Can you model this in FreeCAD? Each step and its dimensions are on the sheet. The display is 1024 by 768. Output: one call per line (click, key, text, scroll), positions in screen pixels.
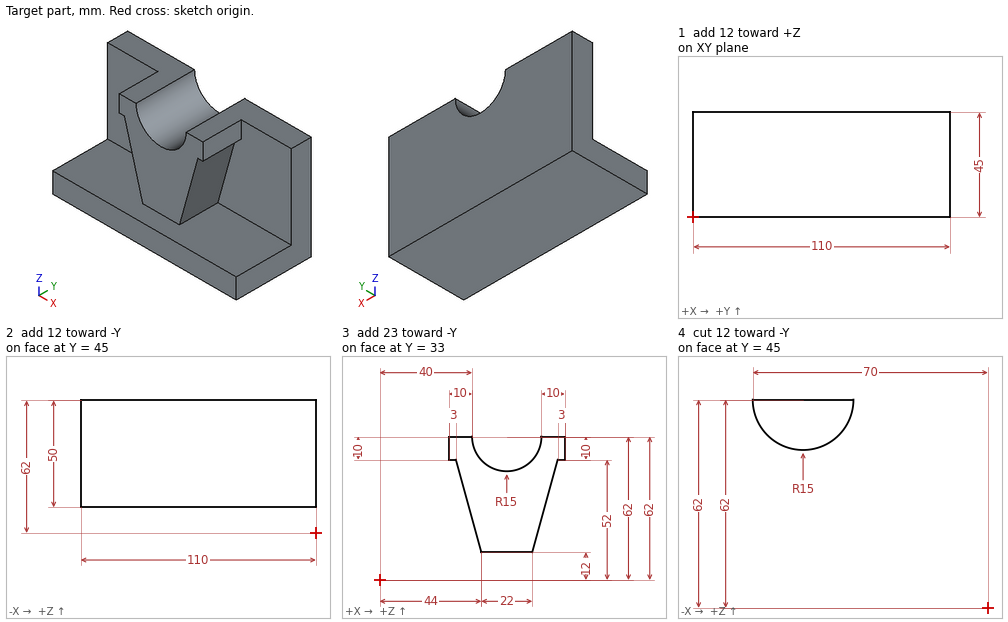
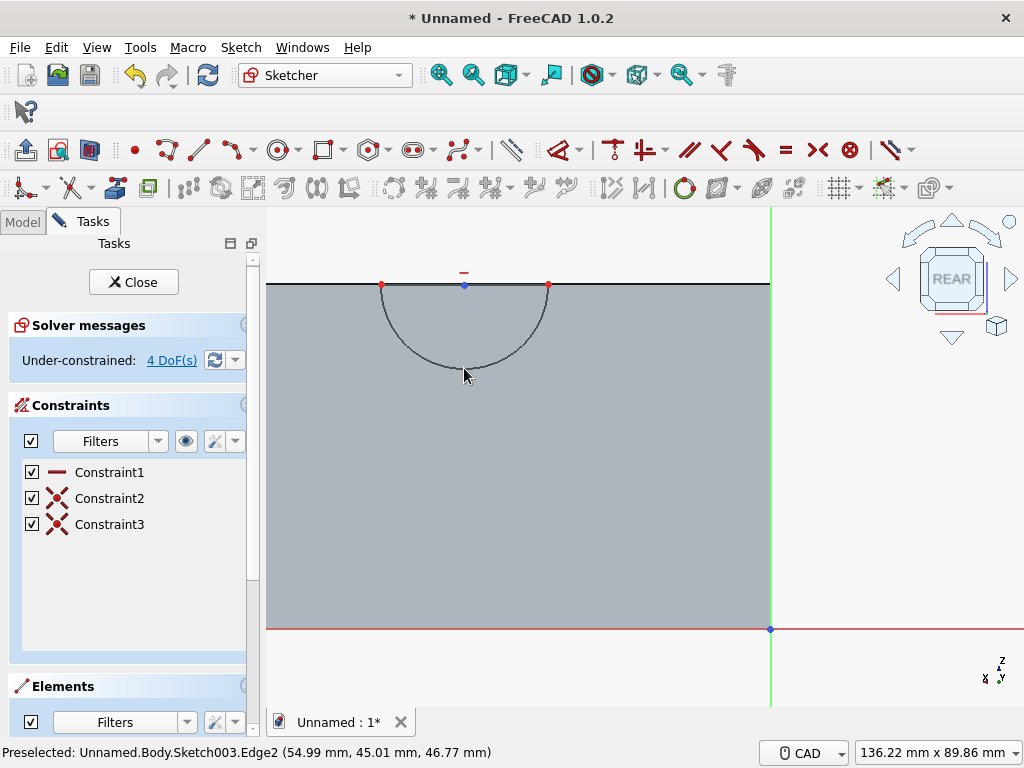
click(558, 150)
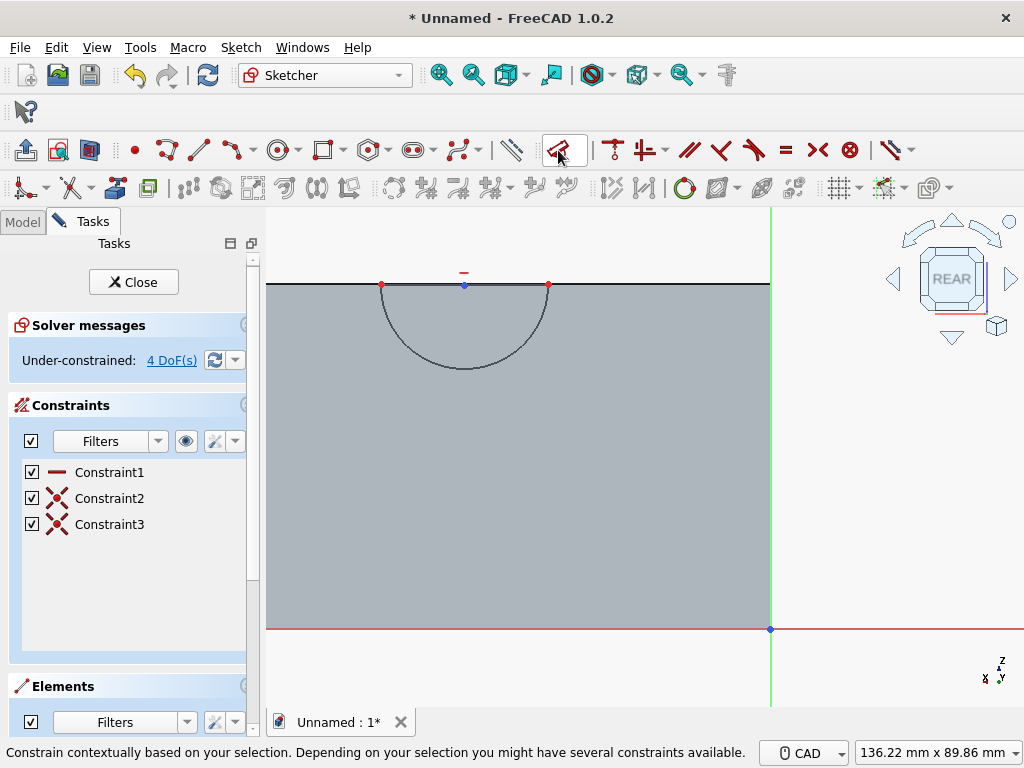
click(415, 353)
click(396, 379)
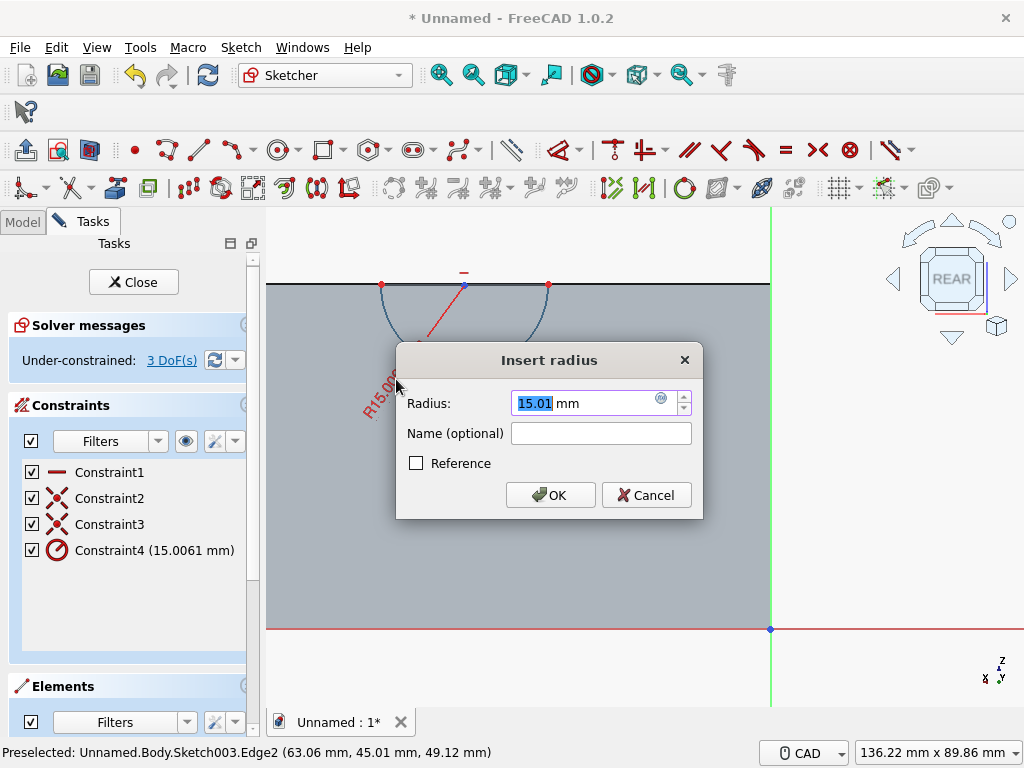
text(15)
key(Return)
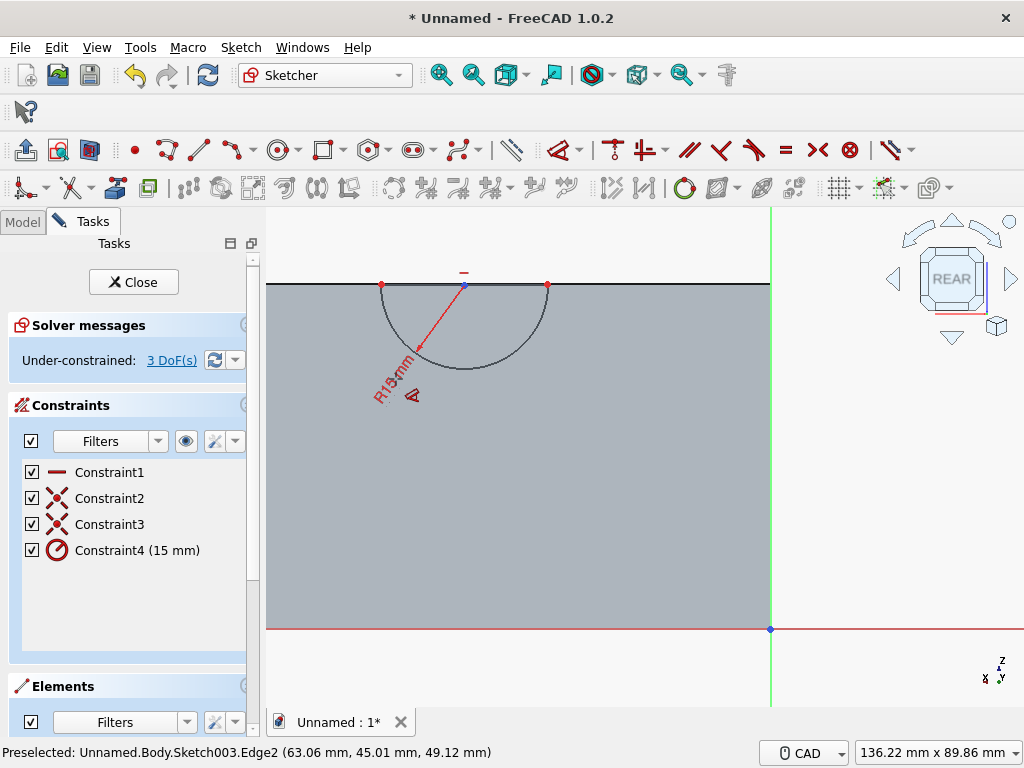
click(381, 285)
click(576, 663)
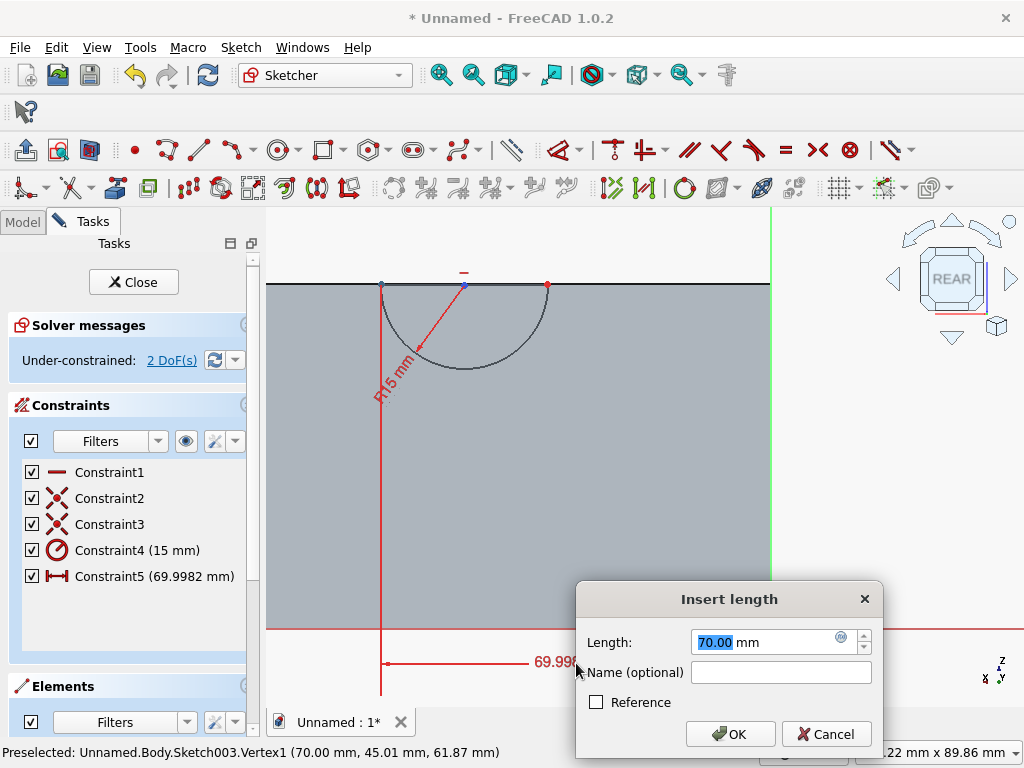
text(70)
key(Return)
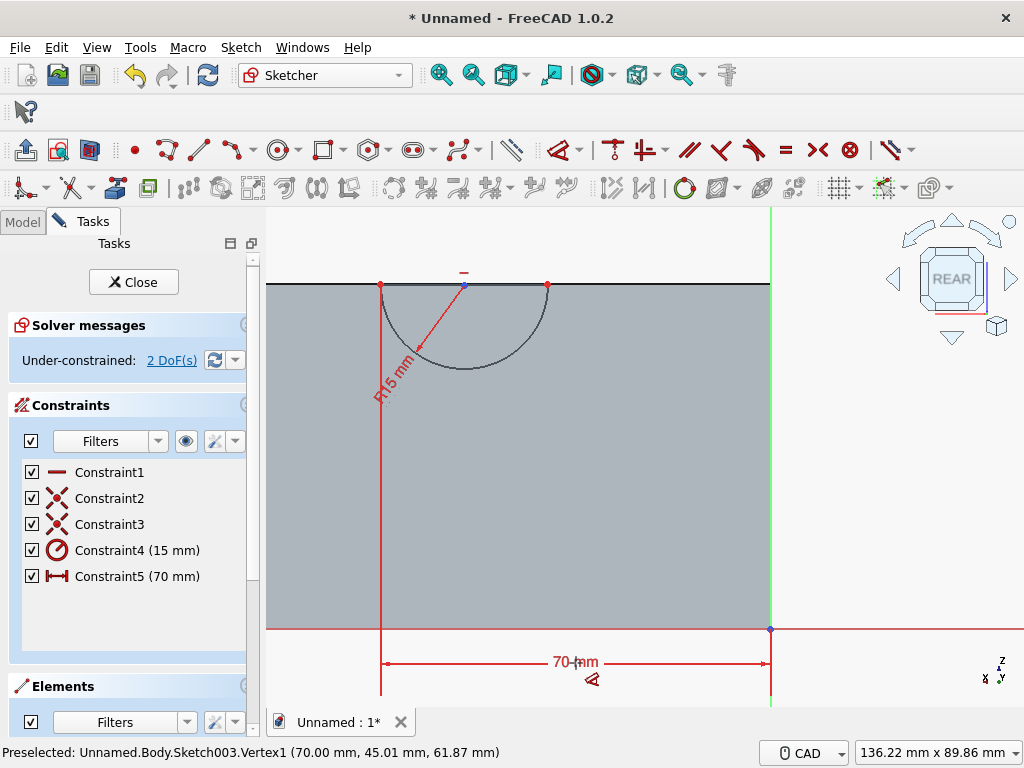
click(381, 285)
click(805, 457)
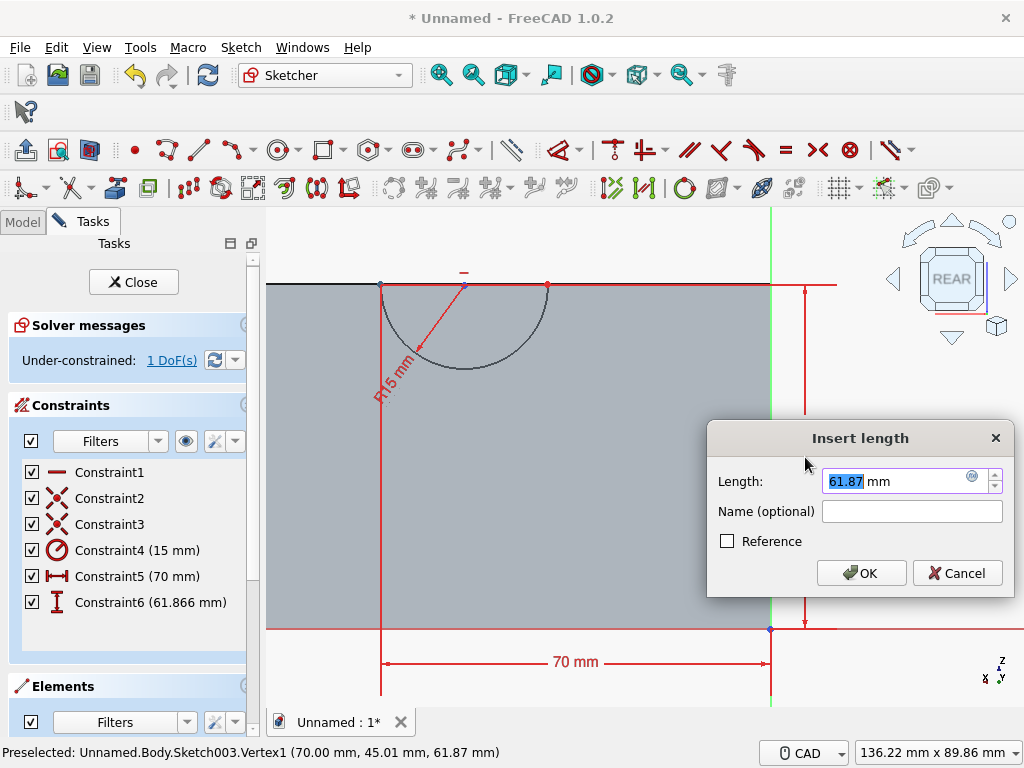
text(62)
key(Return)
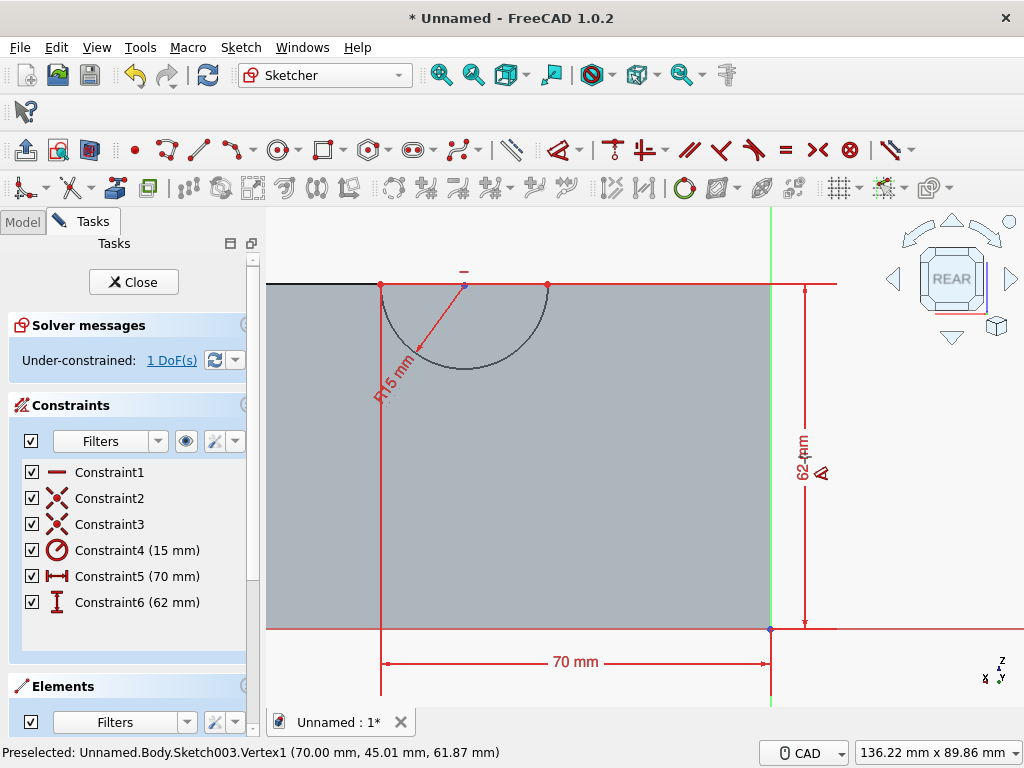
click(464, 285)
click(805, 378)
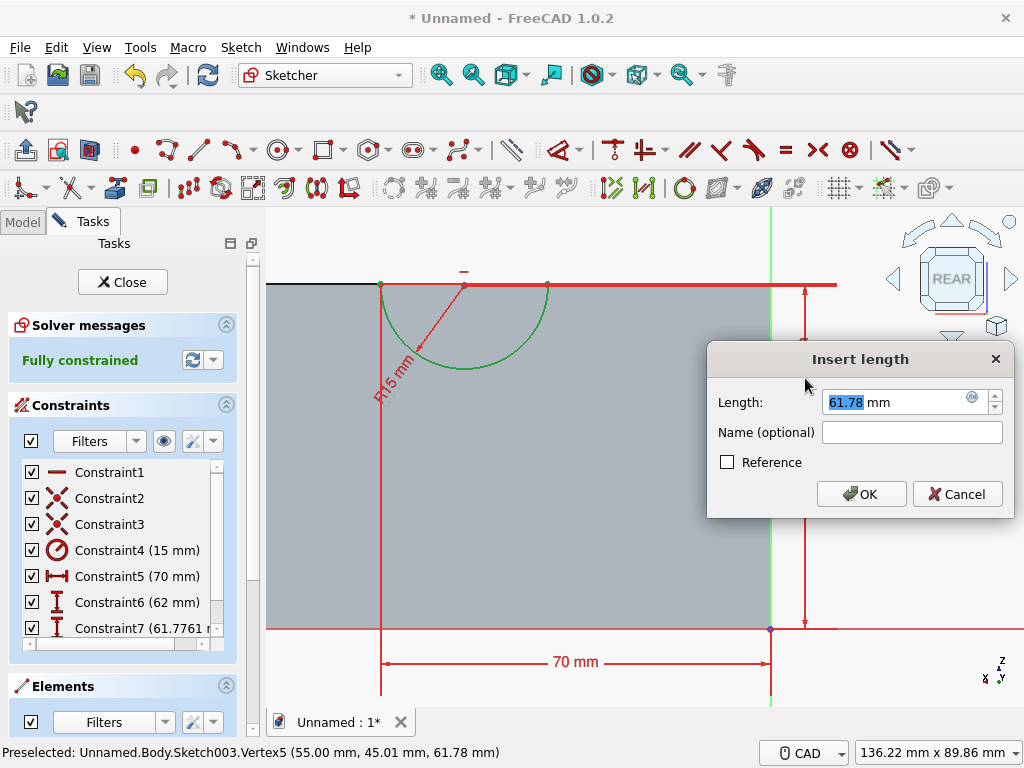
text(62)
key(Return)
key(Escape)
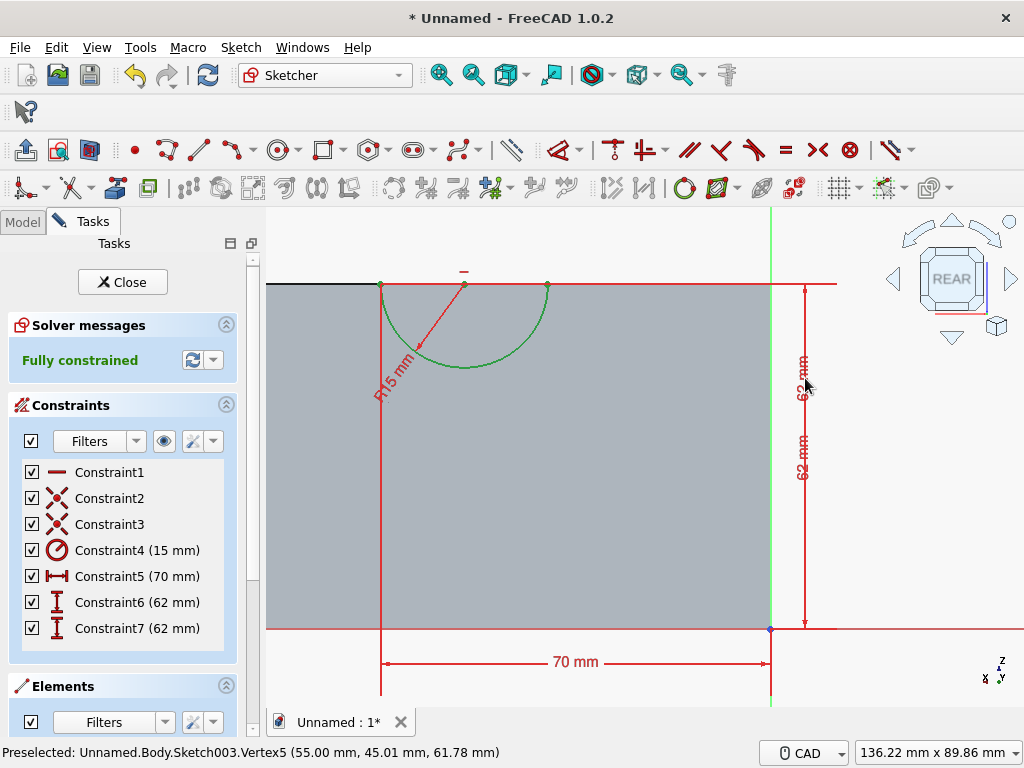
click(123, 282)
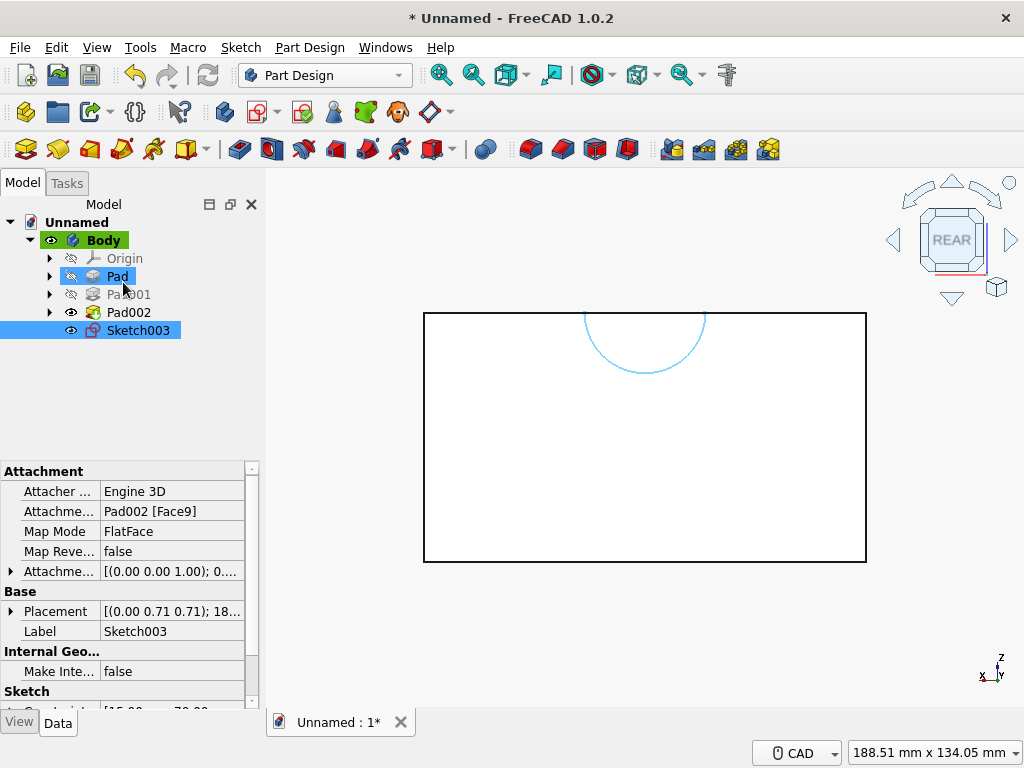
click(240, 150)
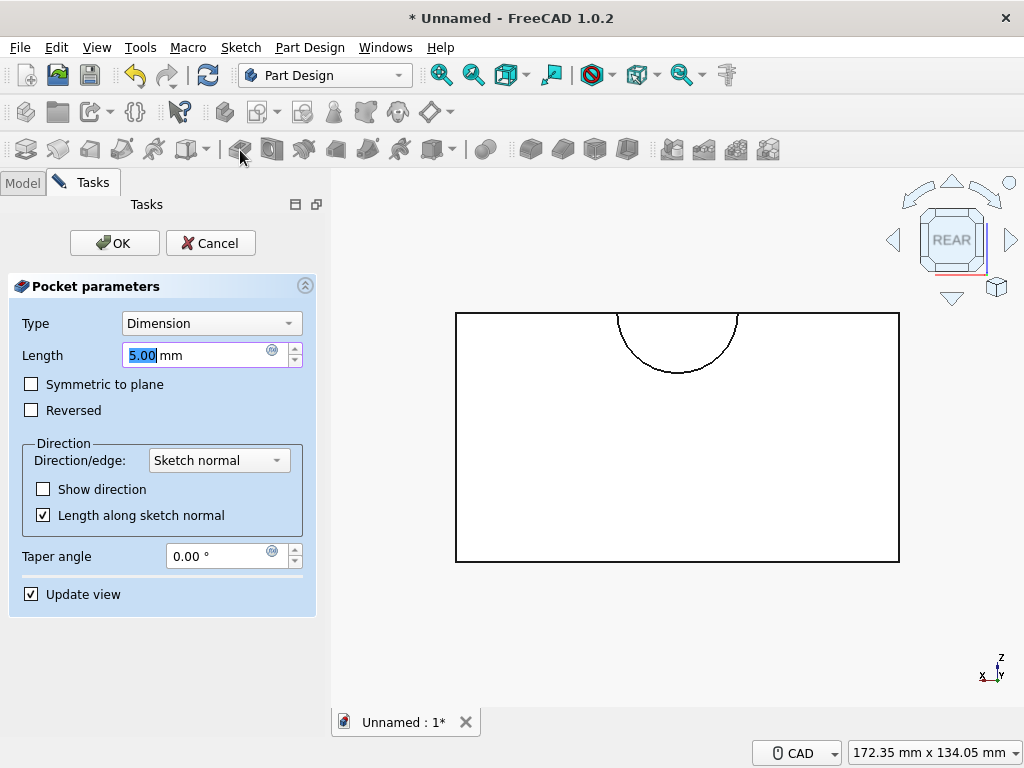
text(12)
key(Tab)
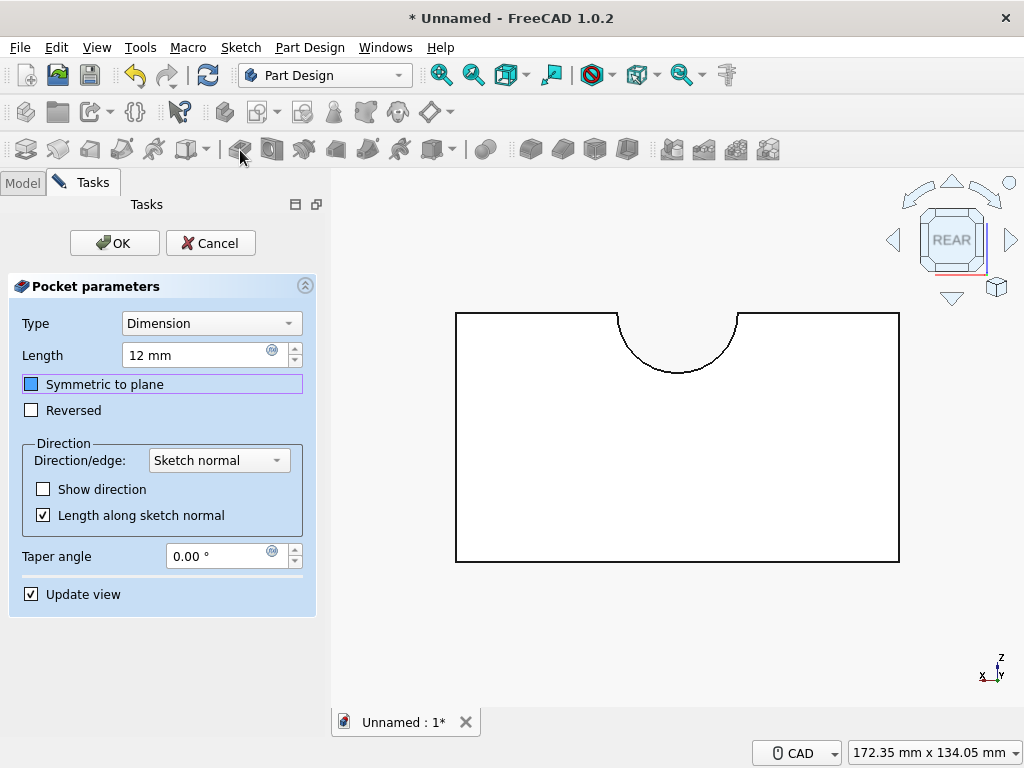
click(115, 243)